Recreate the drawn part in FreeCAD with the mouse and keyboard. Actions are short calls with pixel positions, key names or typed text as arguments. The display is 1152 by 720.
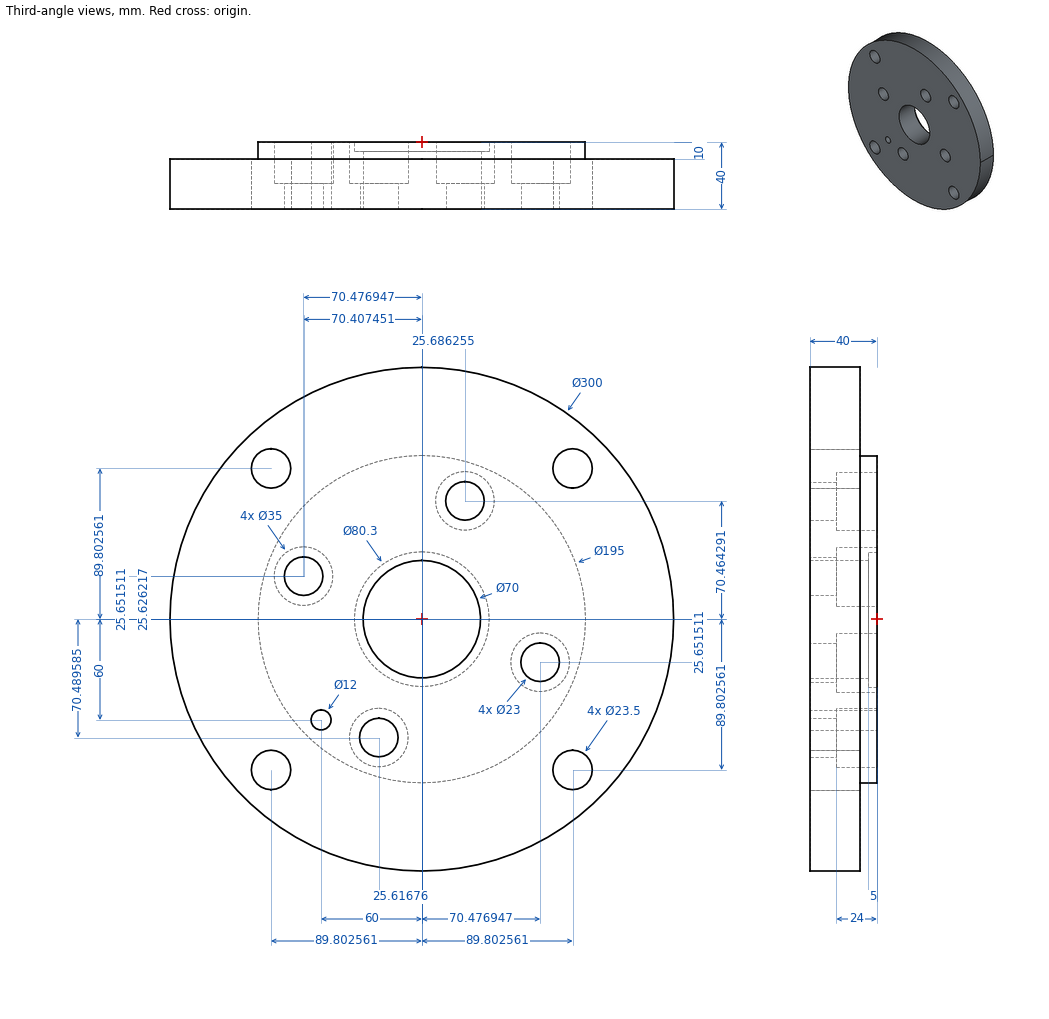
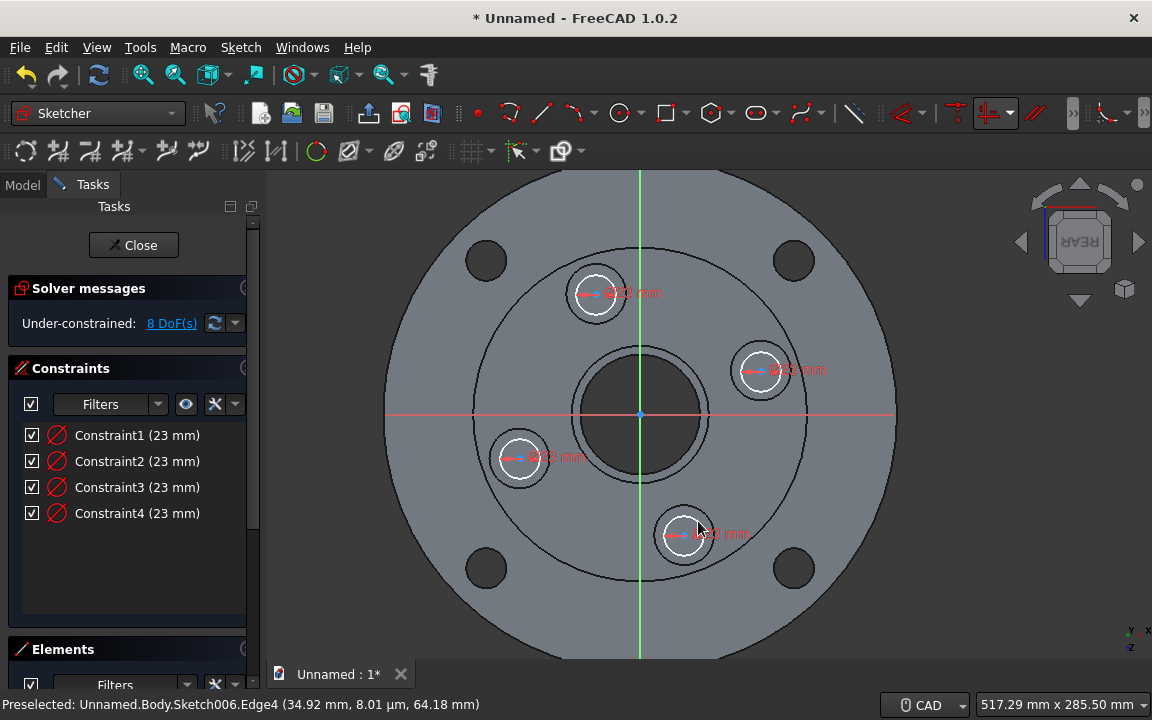
click(902, 114)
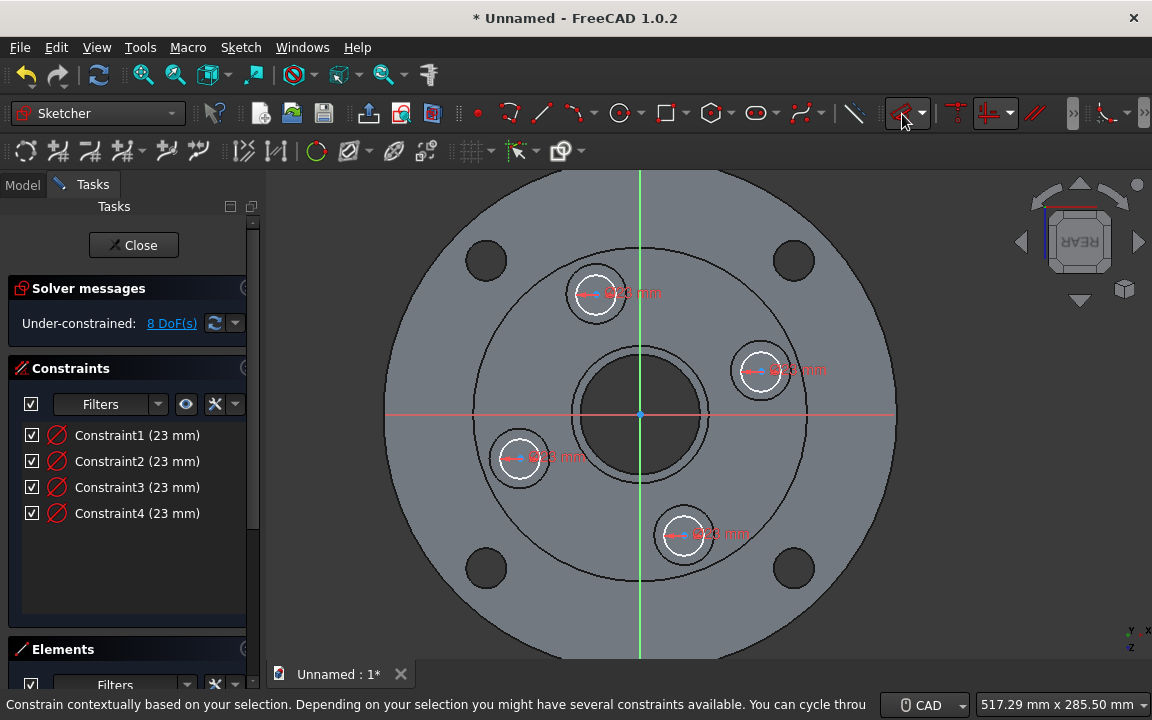
click(596, 295)
click(618, 261)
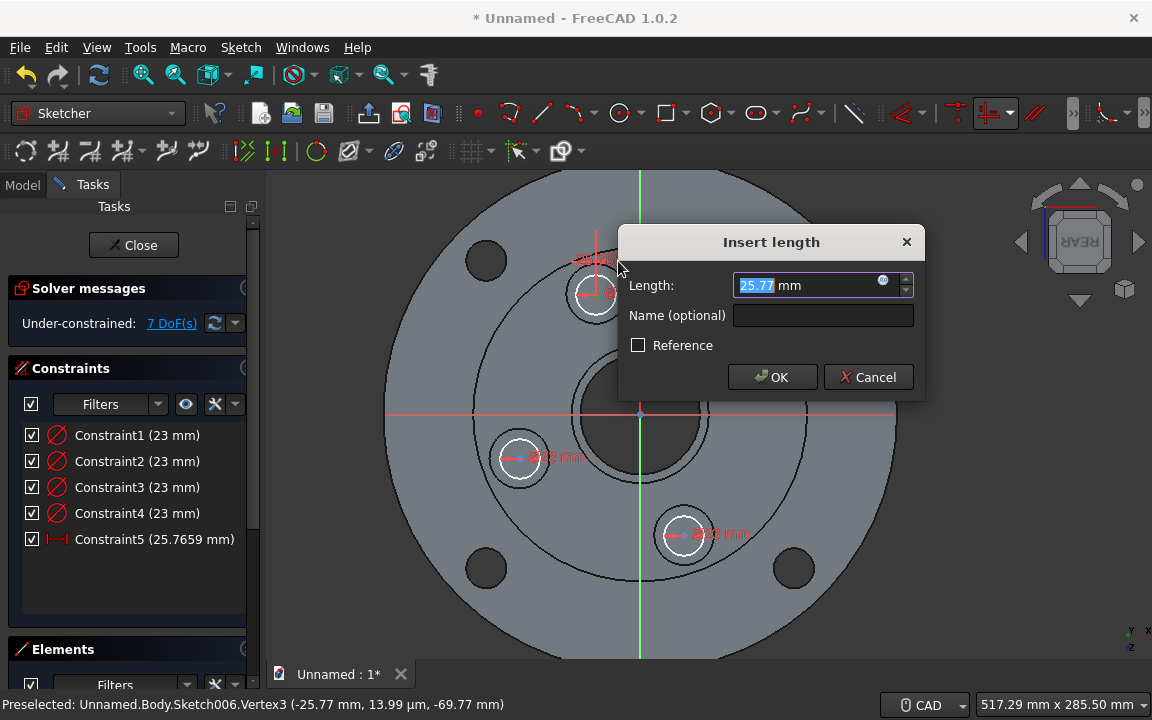
text(25.61676)
key(Return)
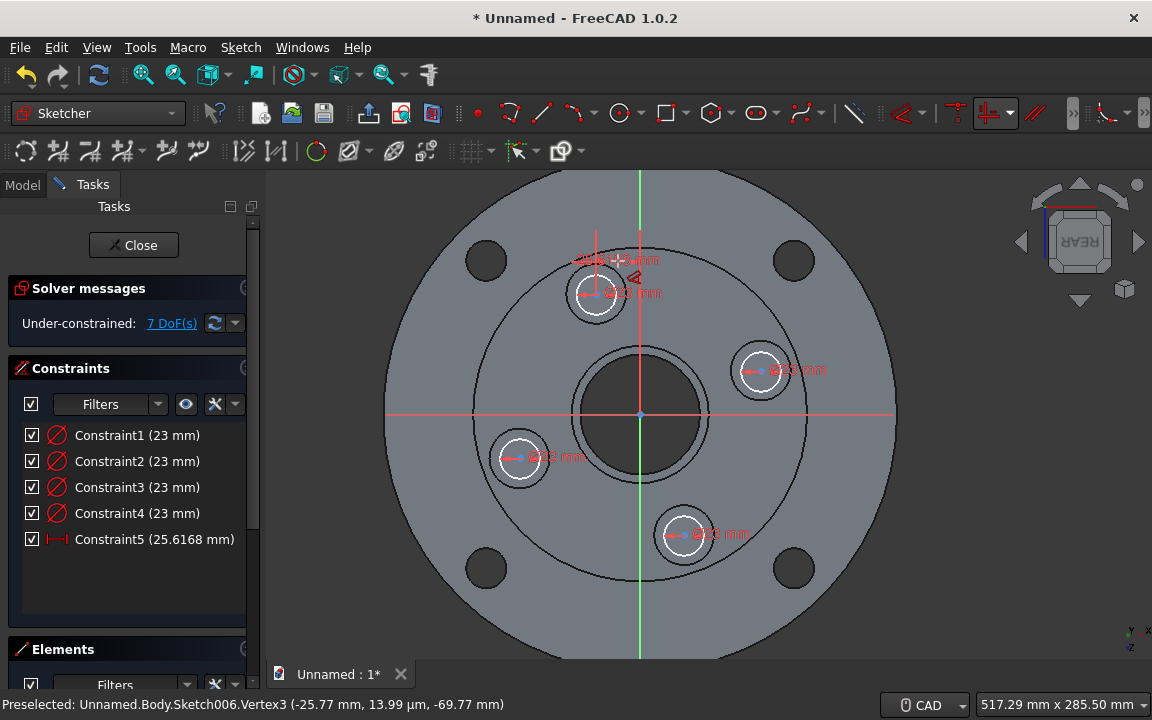
click(761, 372)
click(701, 338)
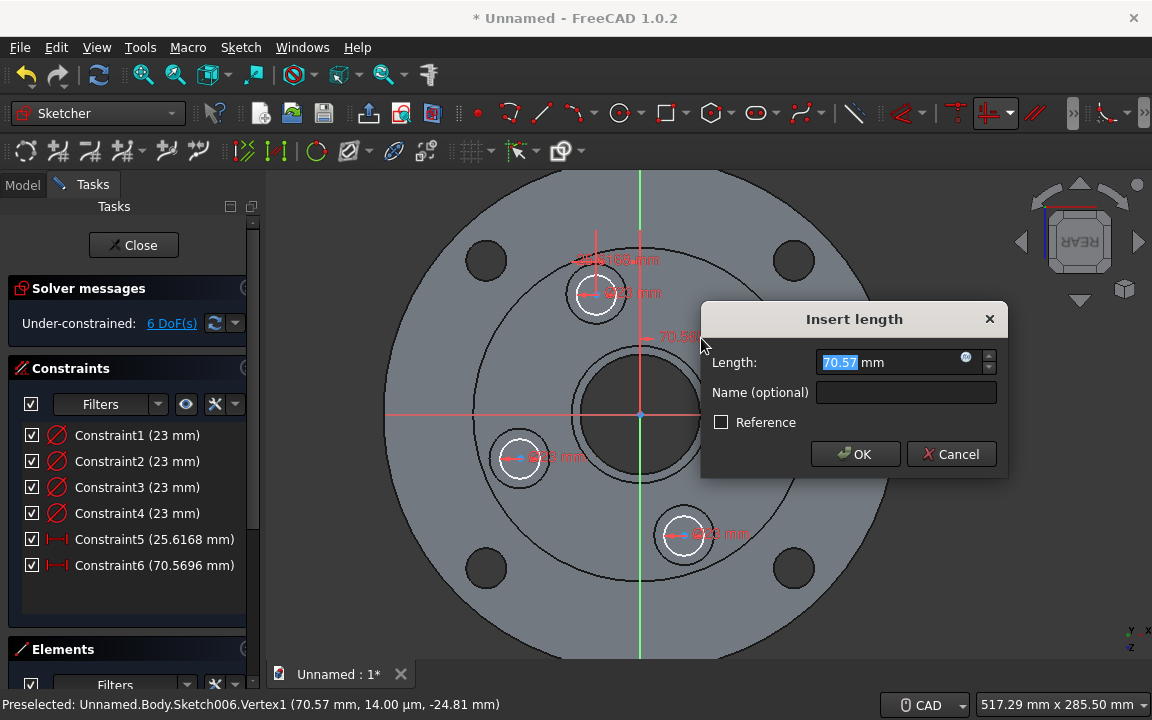
text(70.476947)
key(Return)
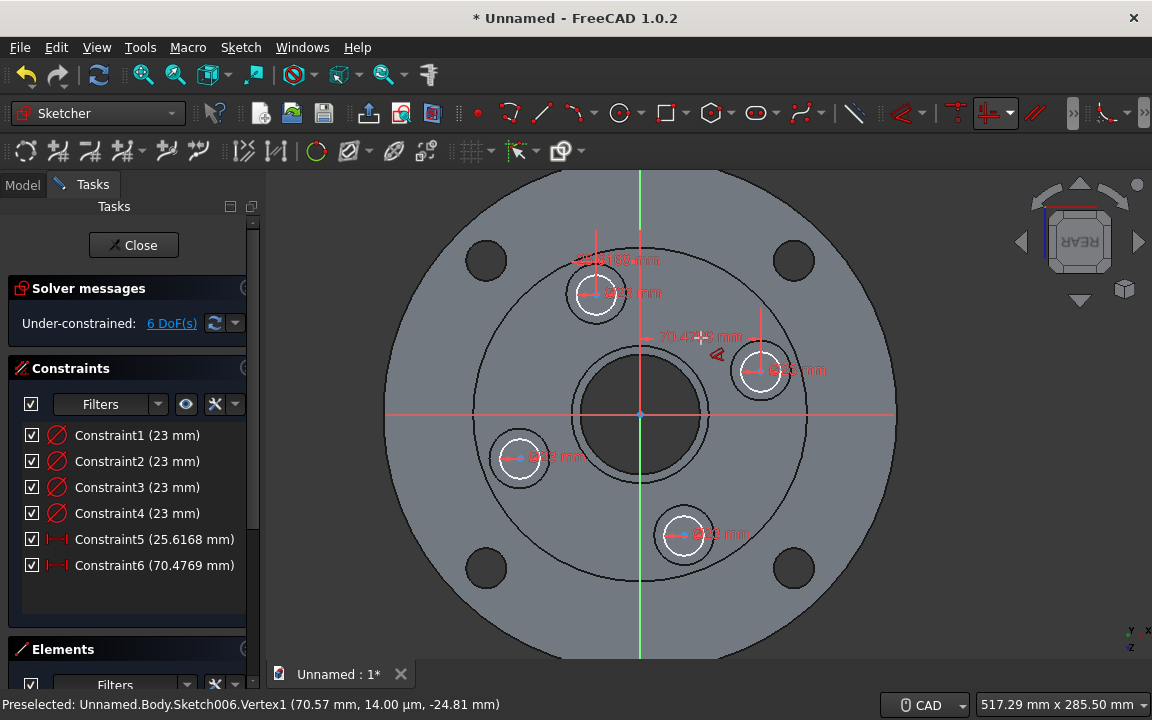
click(761, 372)
click(795, 393)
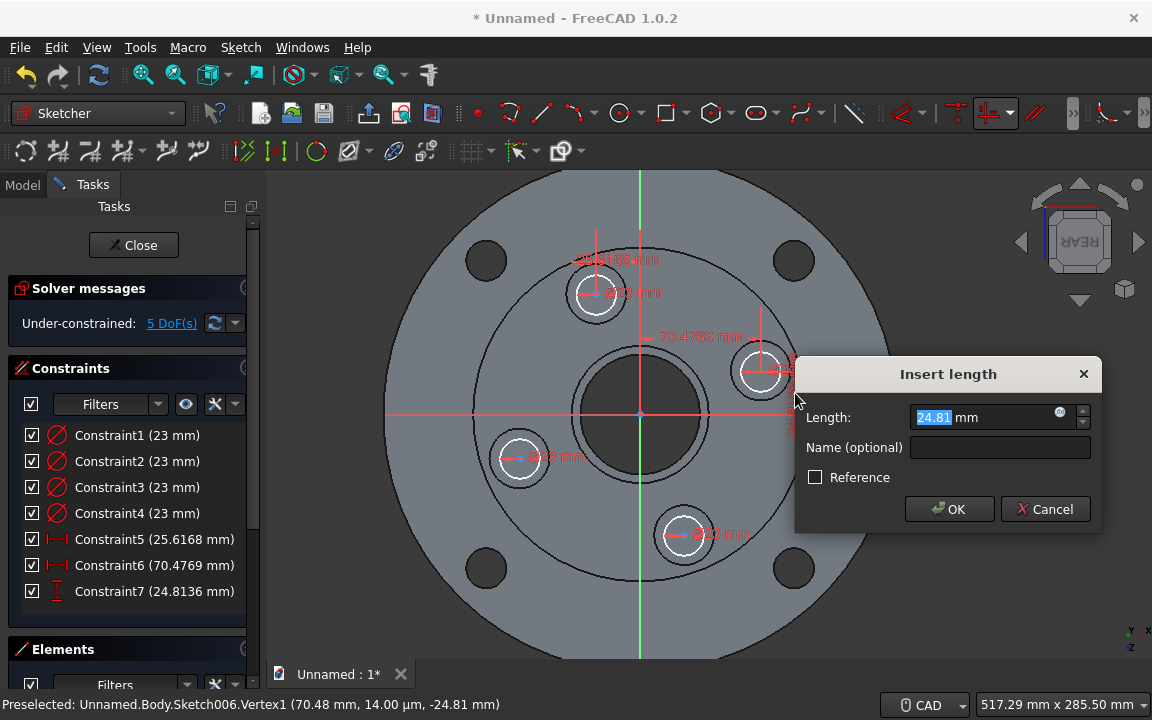
text(25.651511)
key(Return)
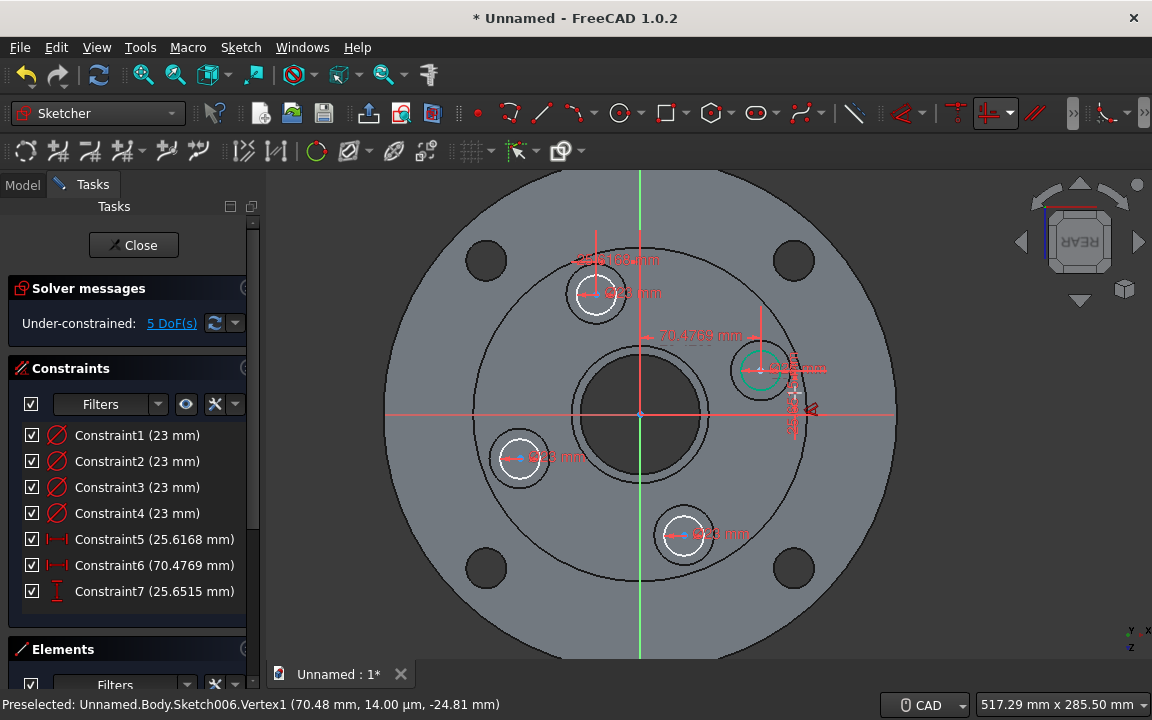
click(520, 459)
click(580, 493)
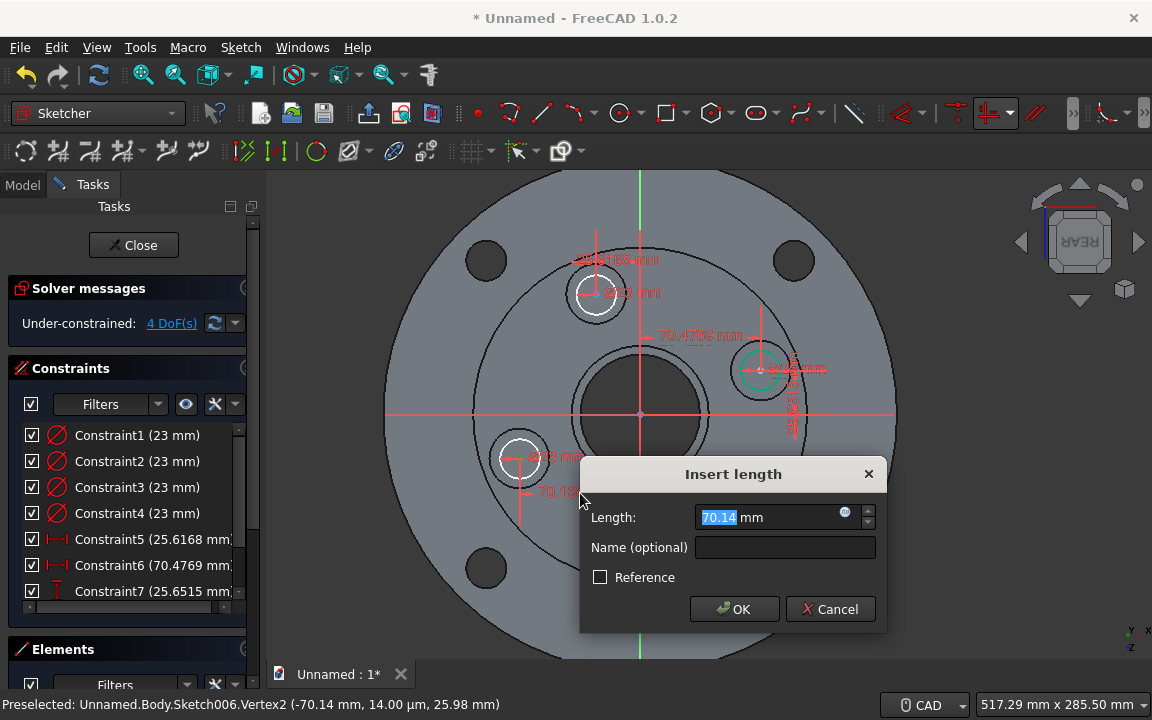
text(70.407451)
key(Return)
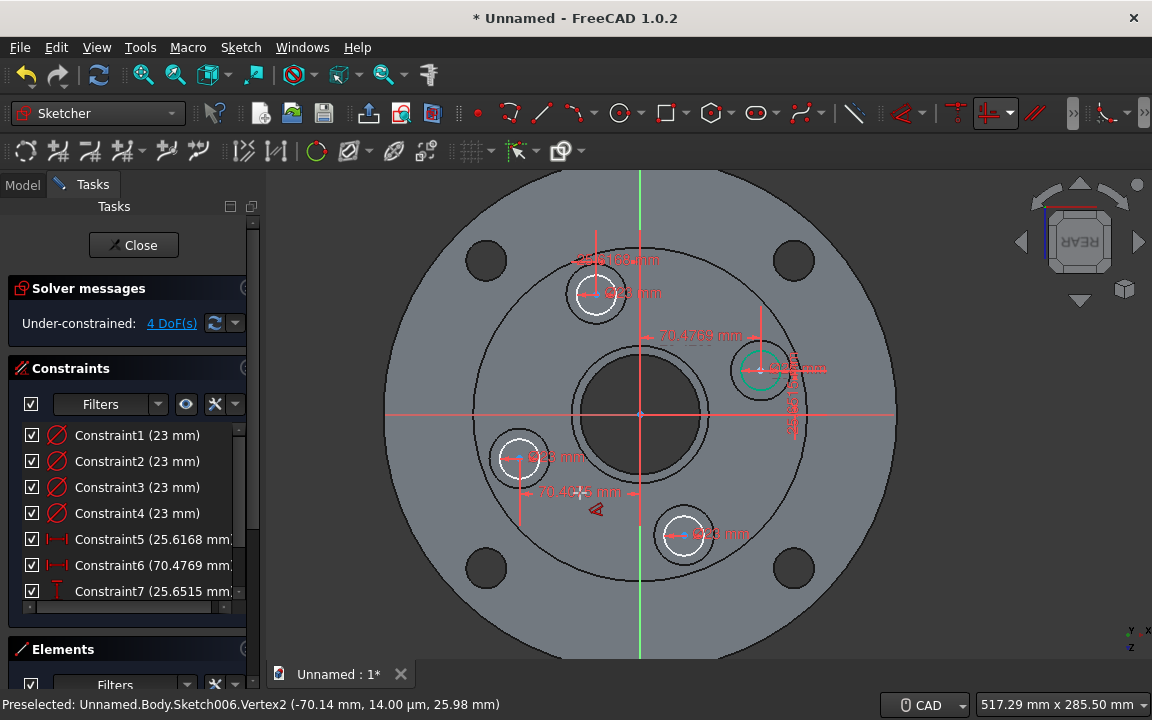
click(520, 459)
click(486, 437)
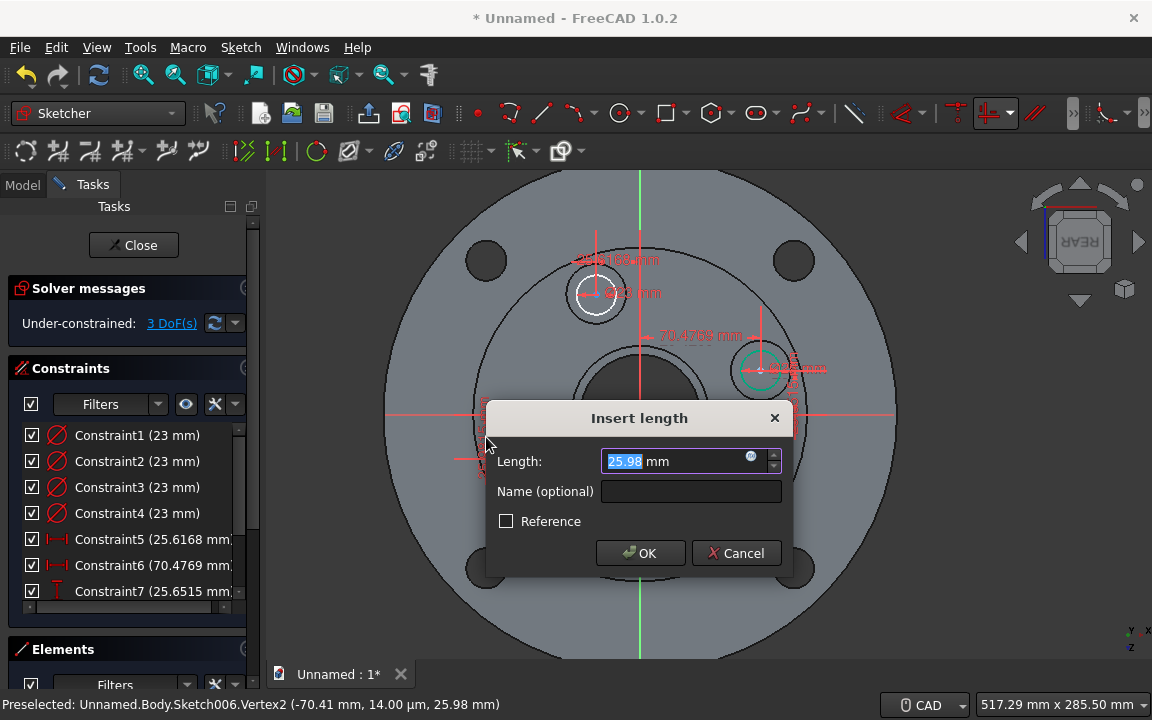
text(25.626217)
key(Return)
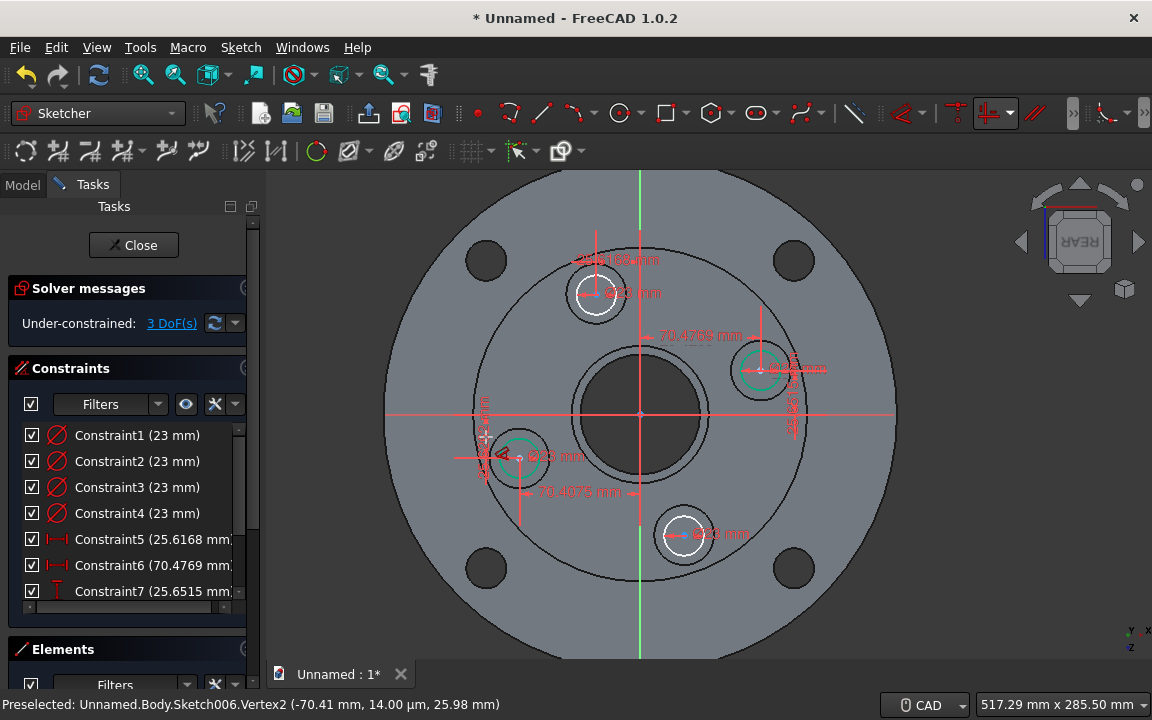
click(596, 295)
click(562, 355)